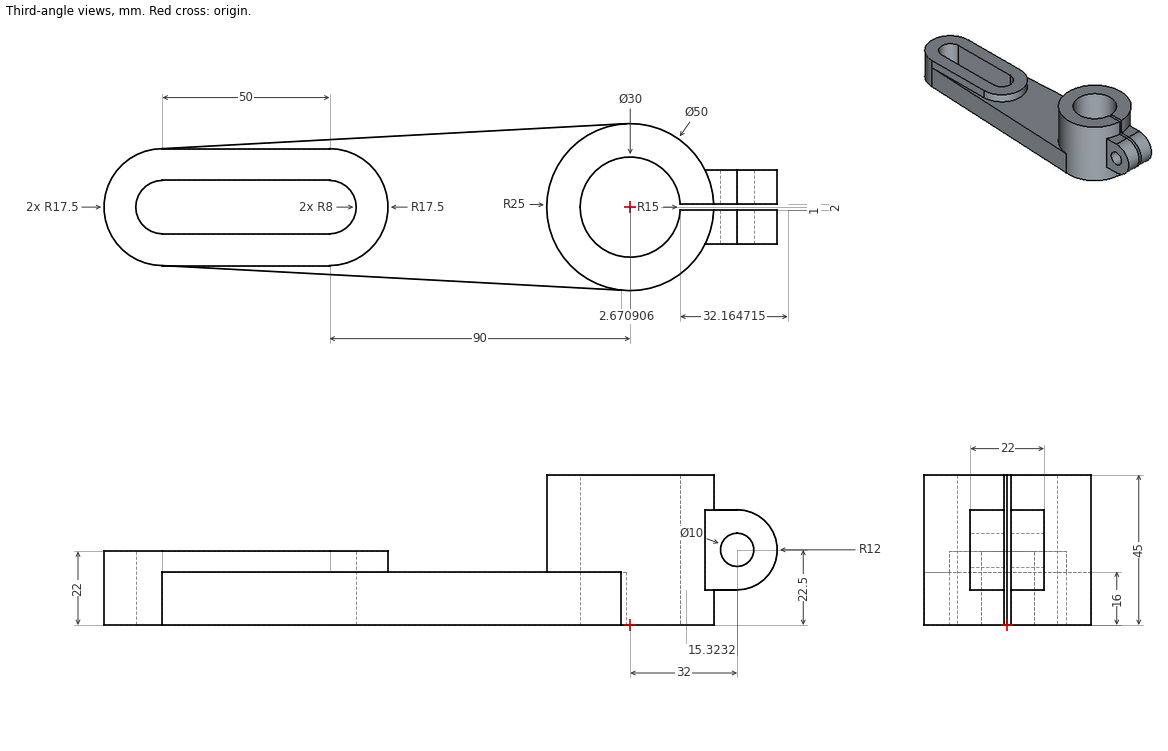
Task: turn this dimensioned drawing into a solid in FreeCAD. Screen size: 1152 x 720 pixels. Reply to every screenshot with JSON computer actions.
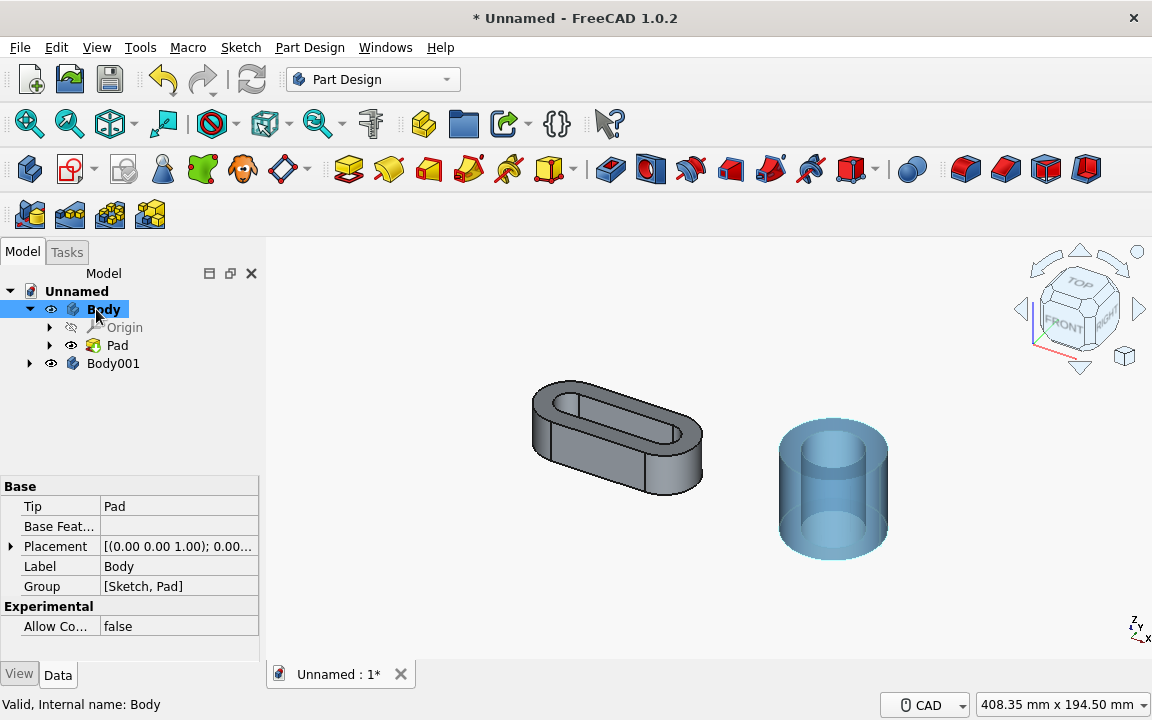
{"action": "left_click", "coordinate": [96, 309]}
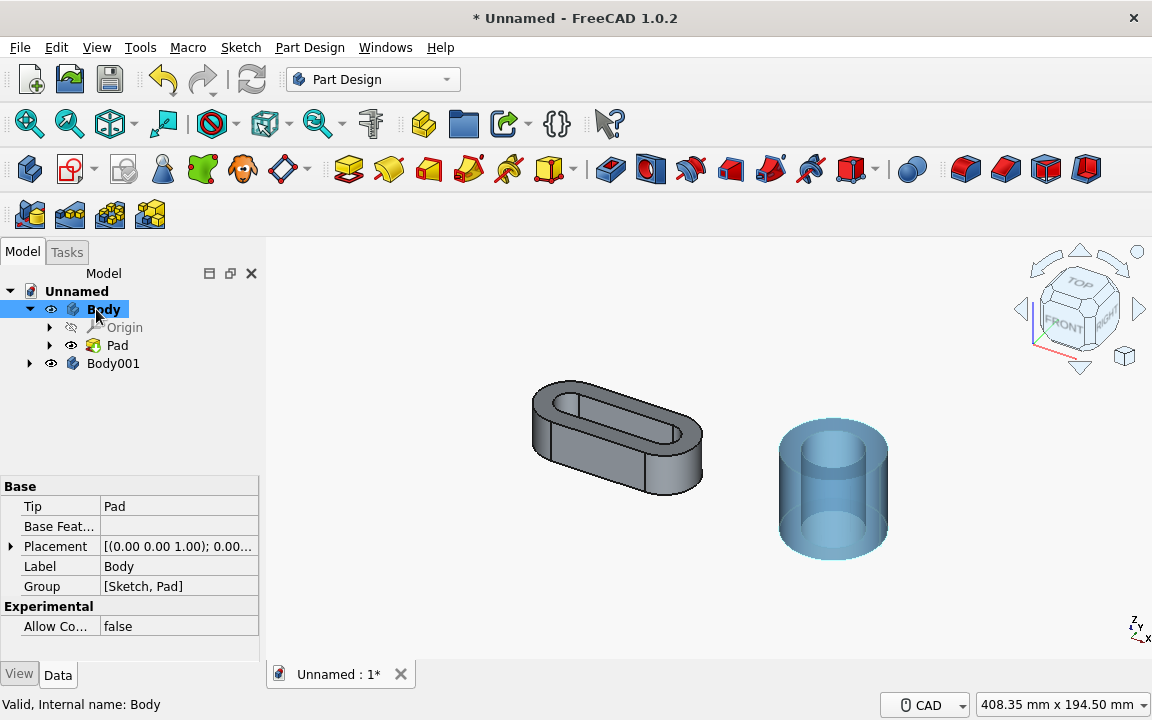
{"action": "left_click", "coordinate": [146, 626]}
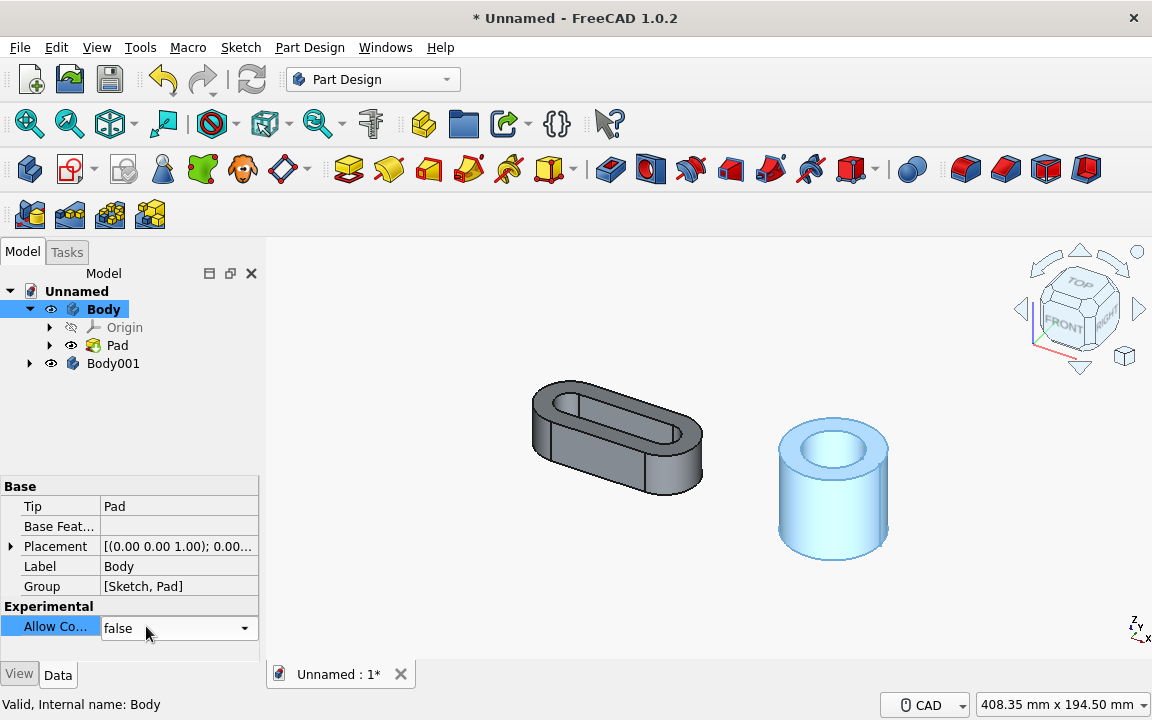
{"action": "left_click", "coordinate": [146, 626]}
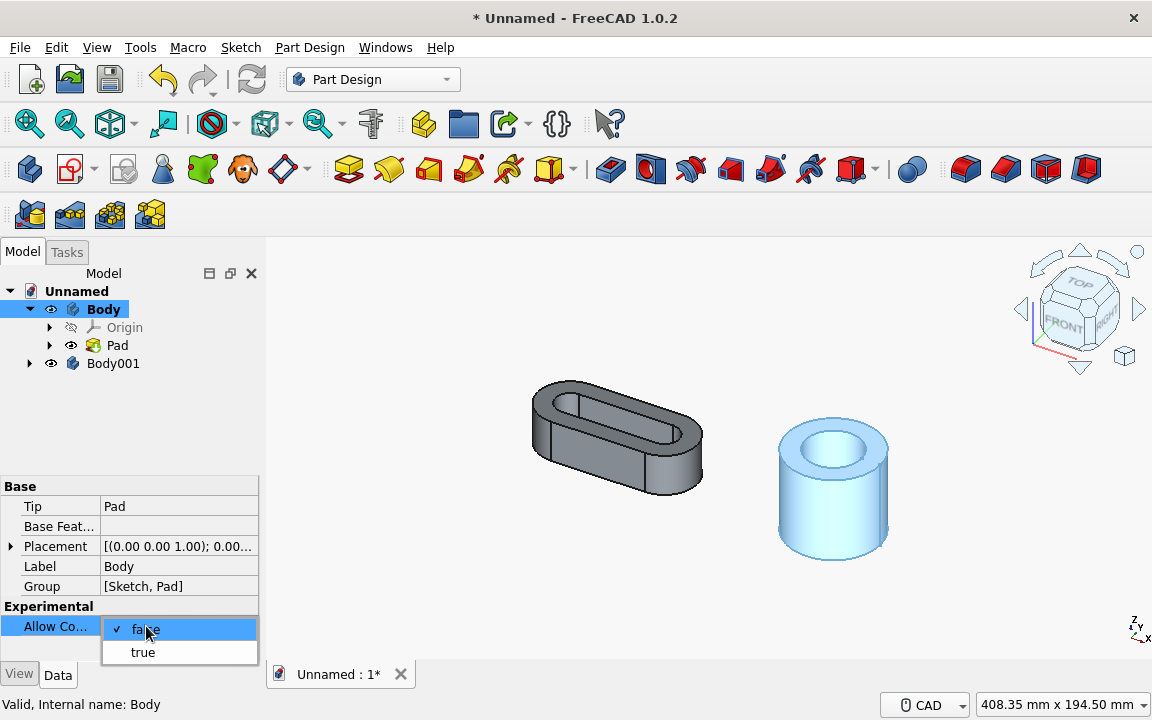
{"action": "left_click", "coordinate": [179, 652]}
{"action": "key", "text": "Return"}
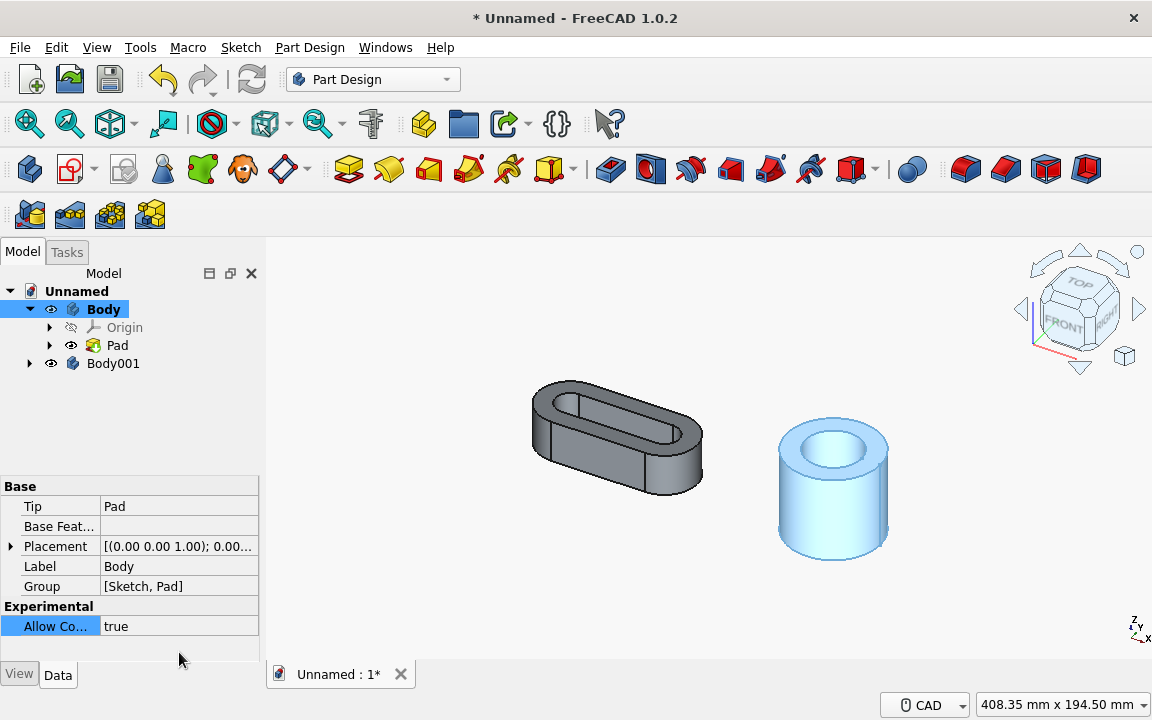
{"action": "left_click", "coordinate": [96, 363]}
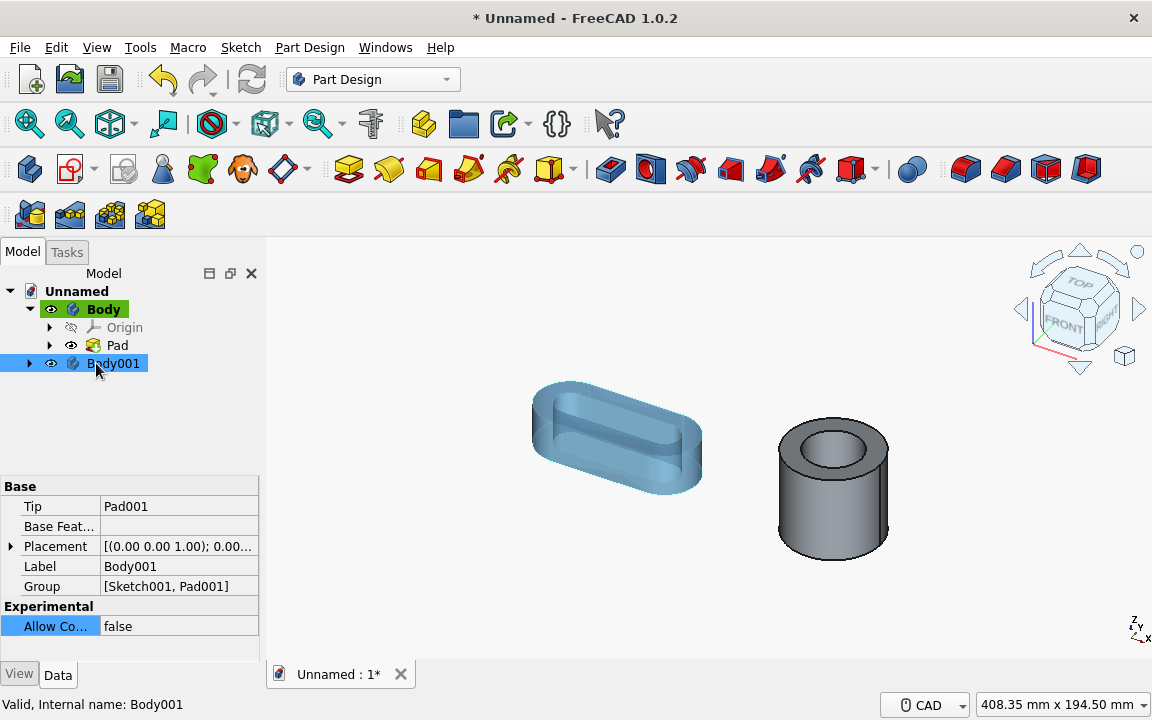
{"action": "left_click", "coordinate": [914, 170]}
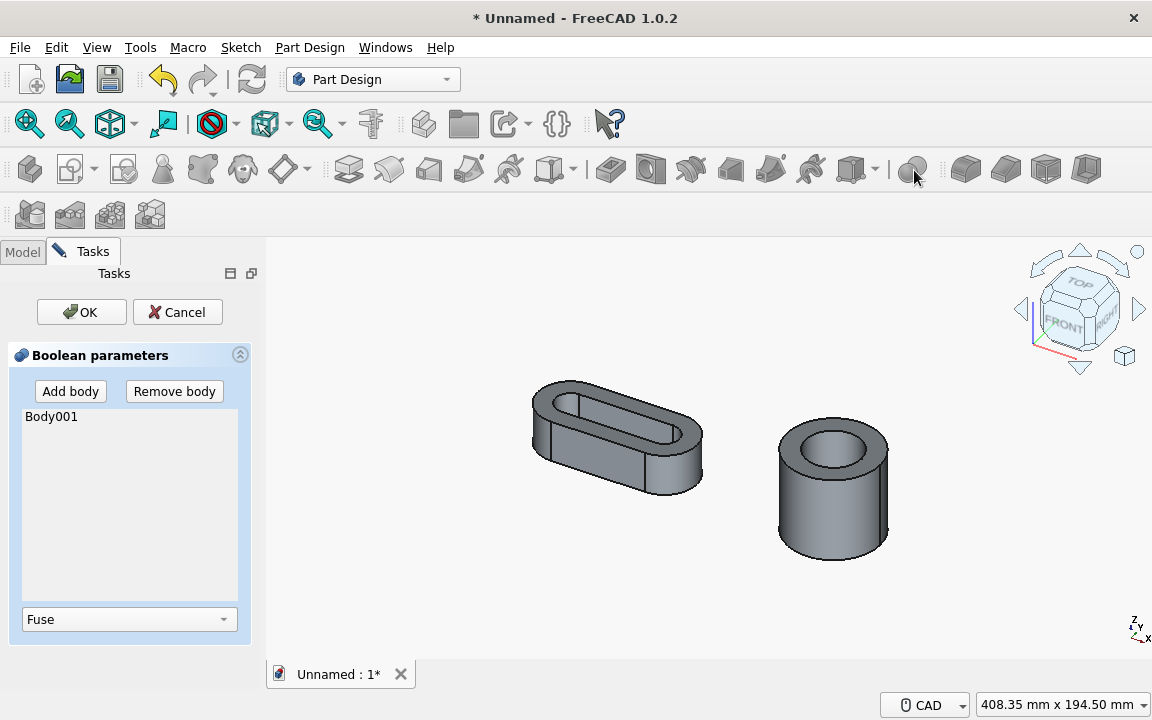
{"action": "left_click", "coordinate": [82, 312]}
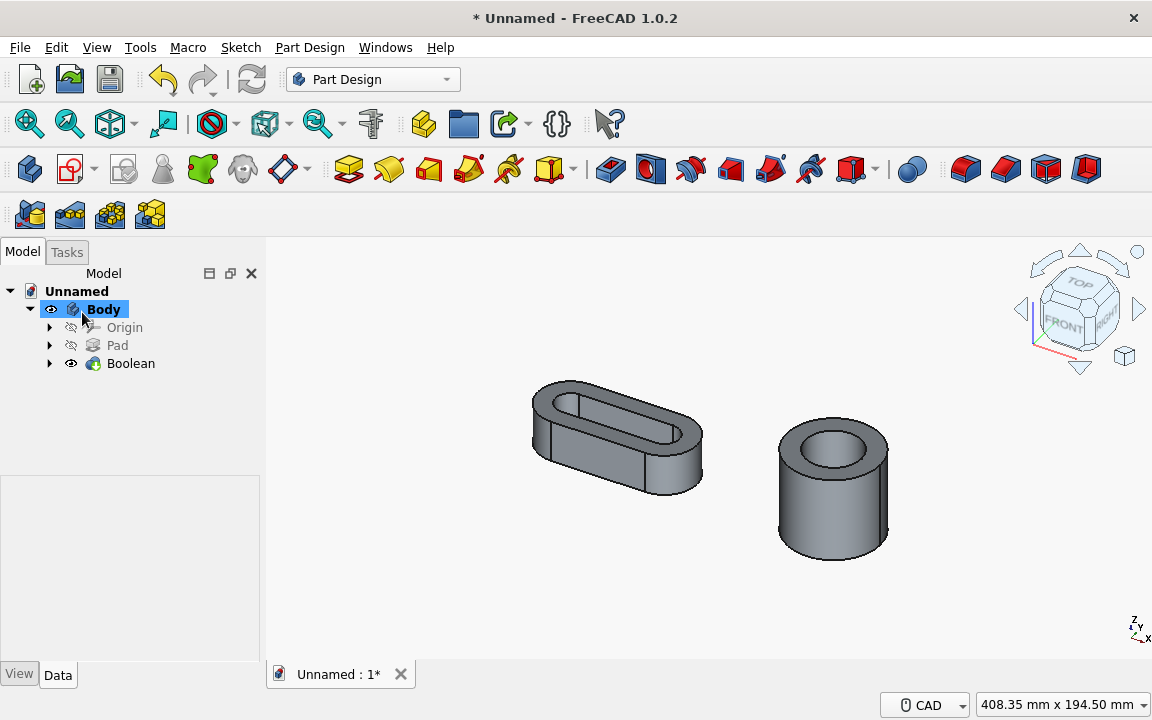
{"action": "left_click", "coordinate": [70, 170]}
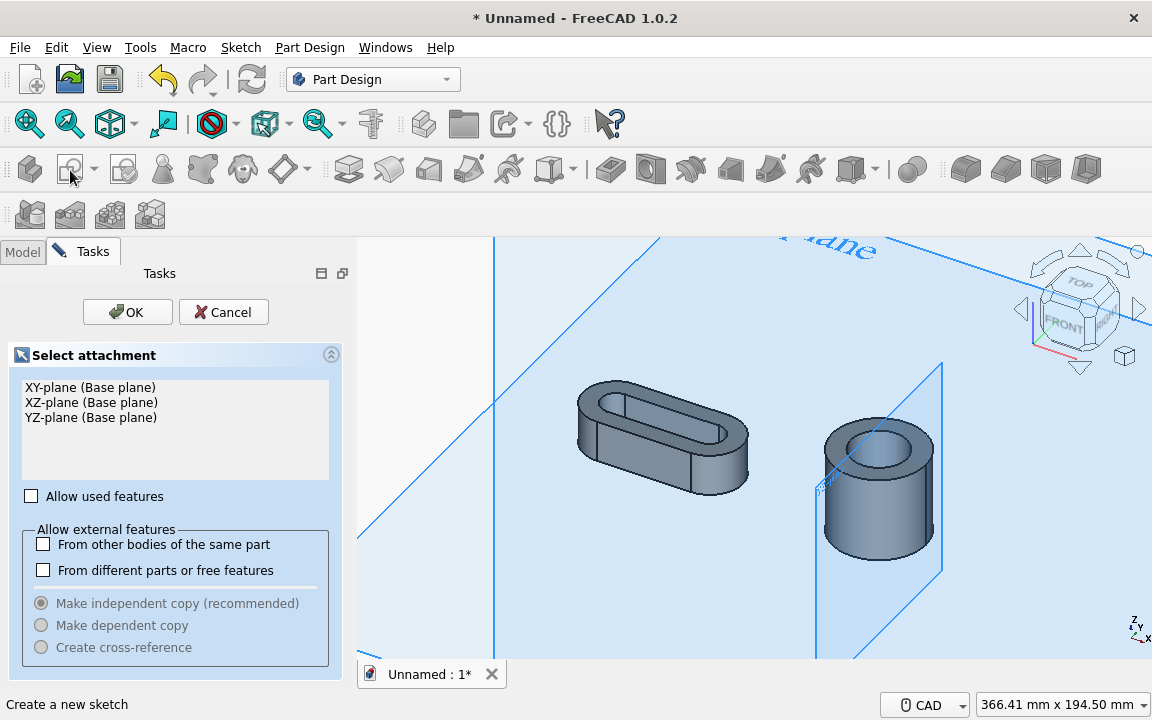
{"action": "left_click", "coordinate": [82, 388]}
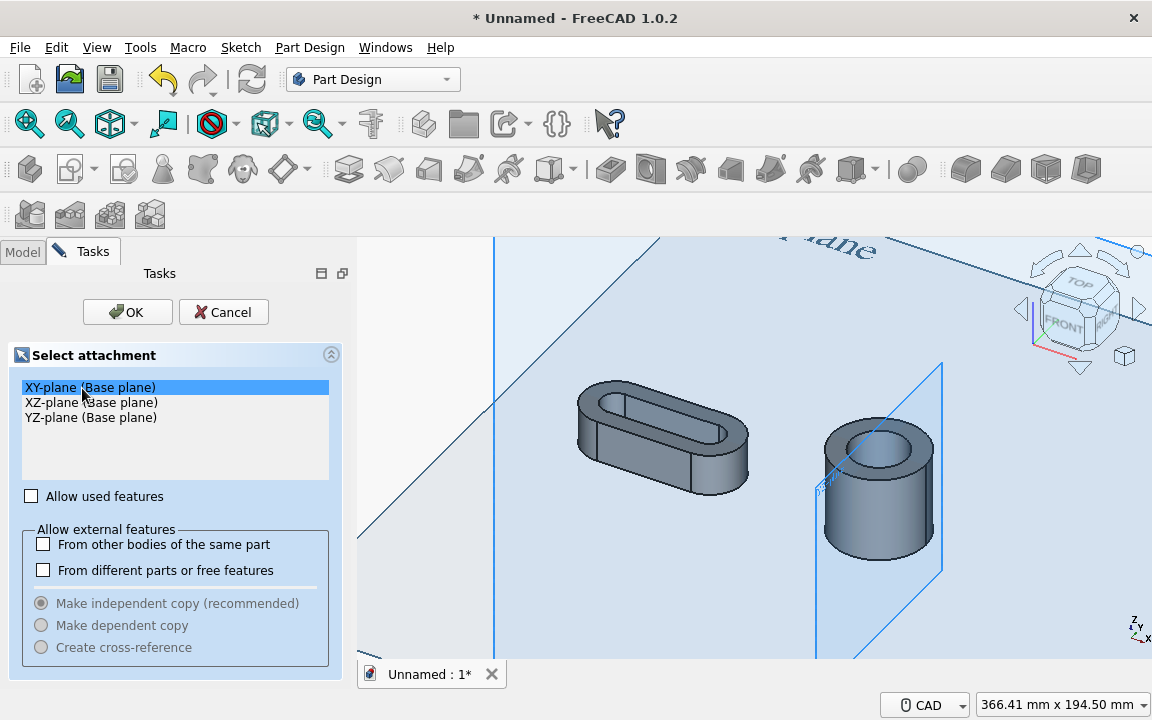
{"action": "left_click", "coordinate": [128, 312]}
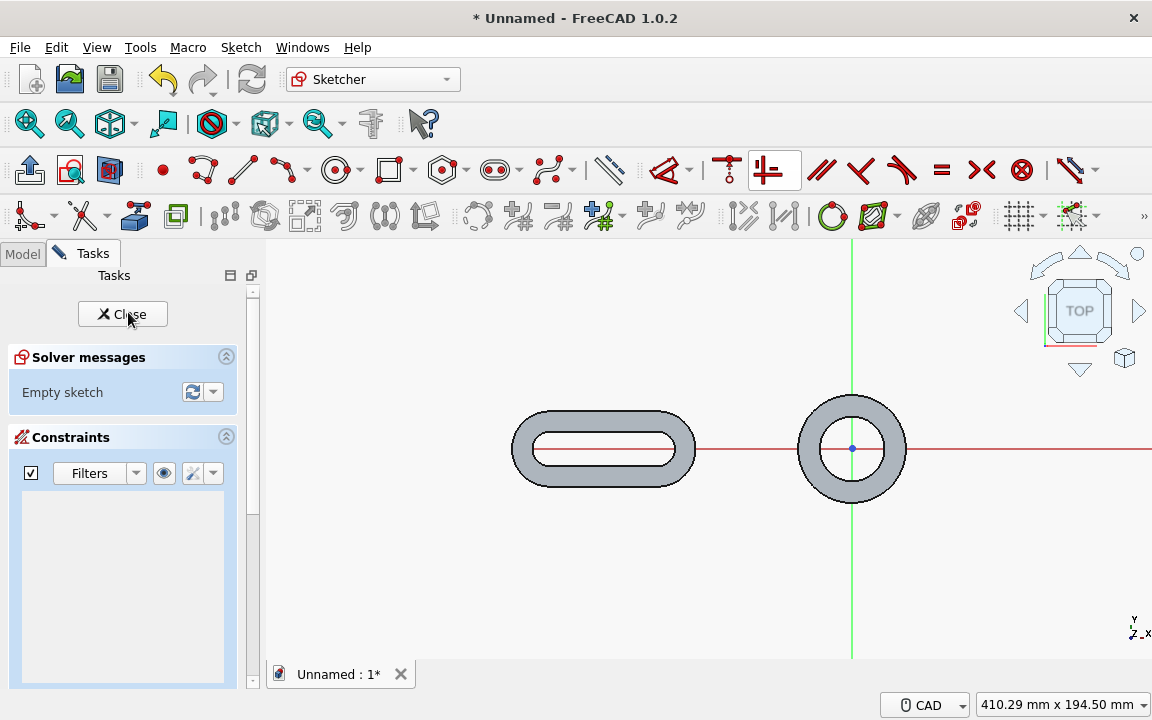
{"action": "left_click", "coordinate": [110, 170]}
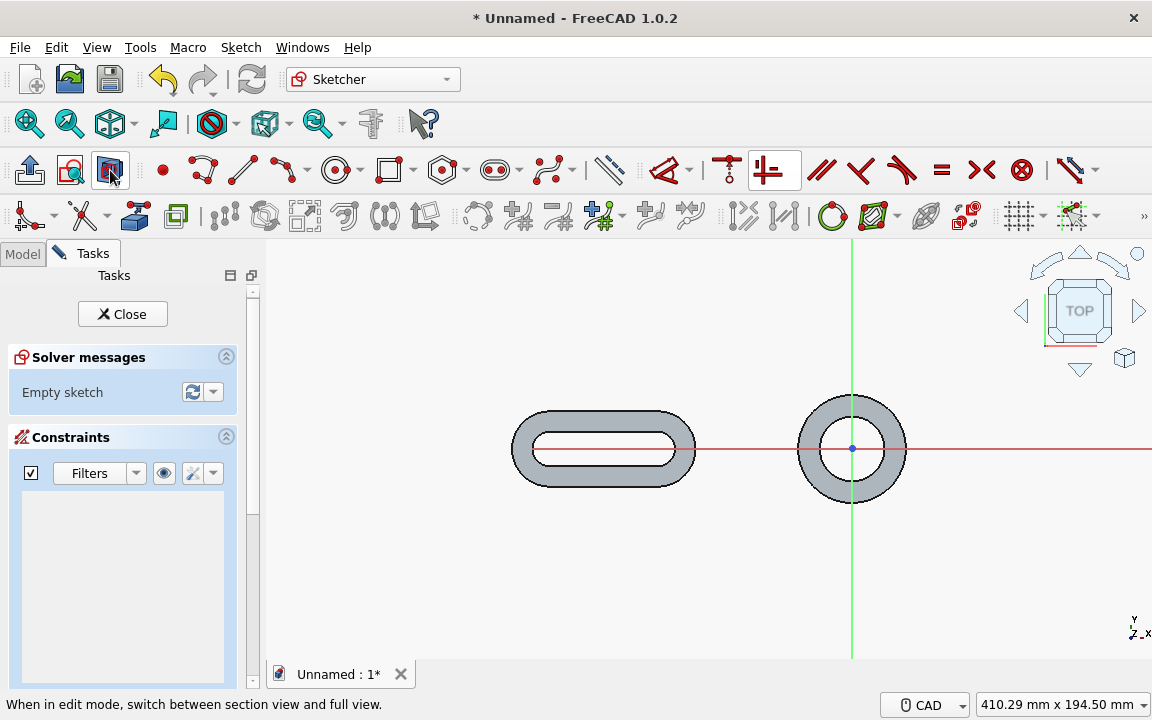
{"action": "scroll", "coordinate": [824, 449], "scroll_direction": "up", "scroll_amount": 2}